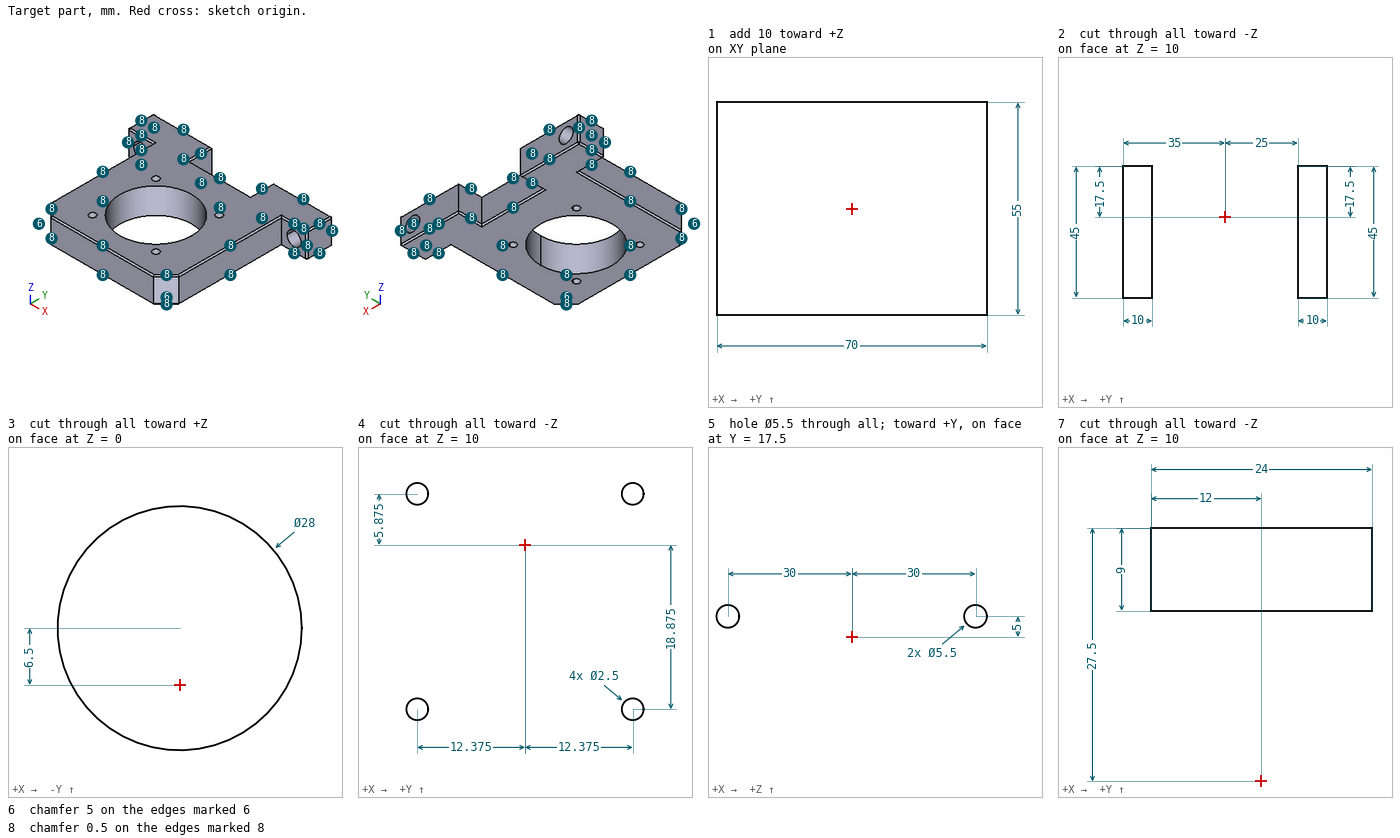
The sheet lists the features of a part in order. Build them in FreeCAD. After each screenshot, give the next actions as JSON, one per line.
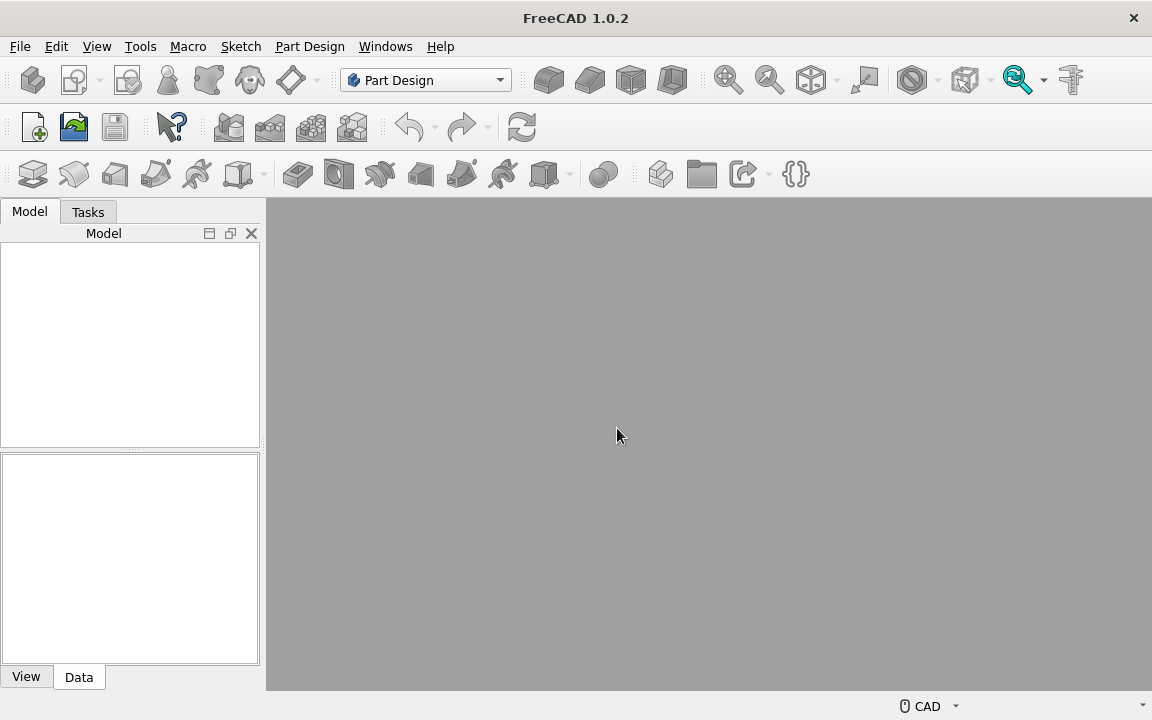
{"action": "left_click", "coordinate": [33, 128]}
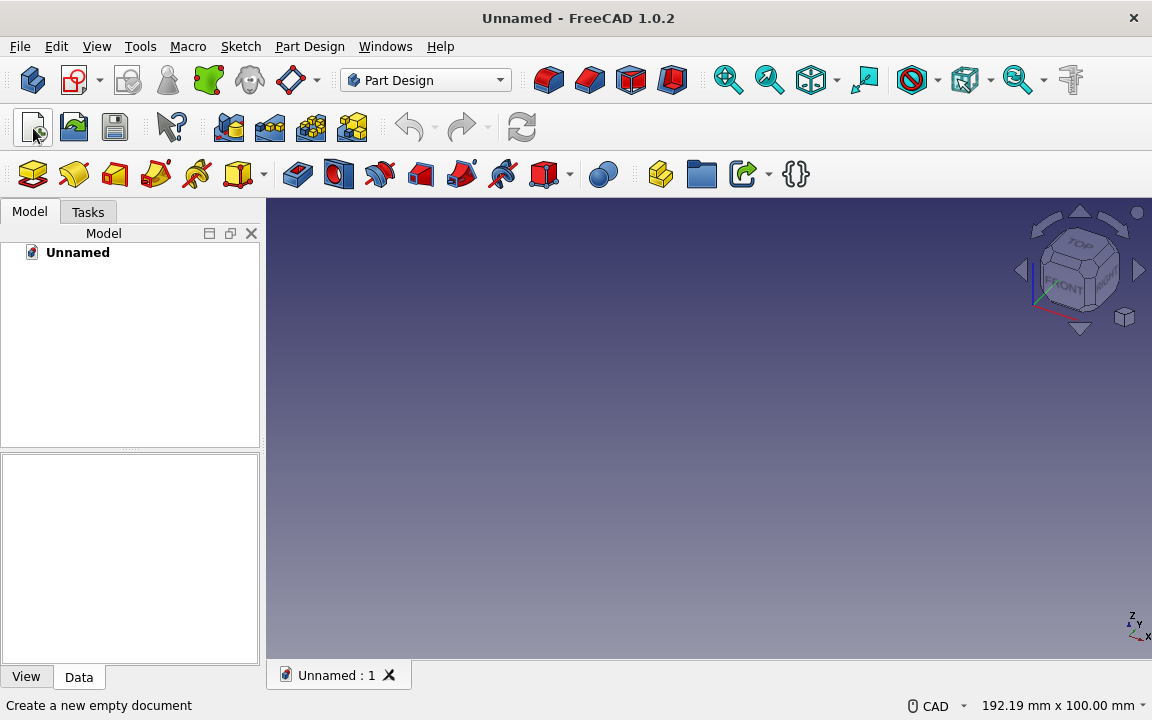
{"action": "left_click", "coordinate": [74, 80]}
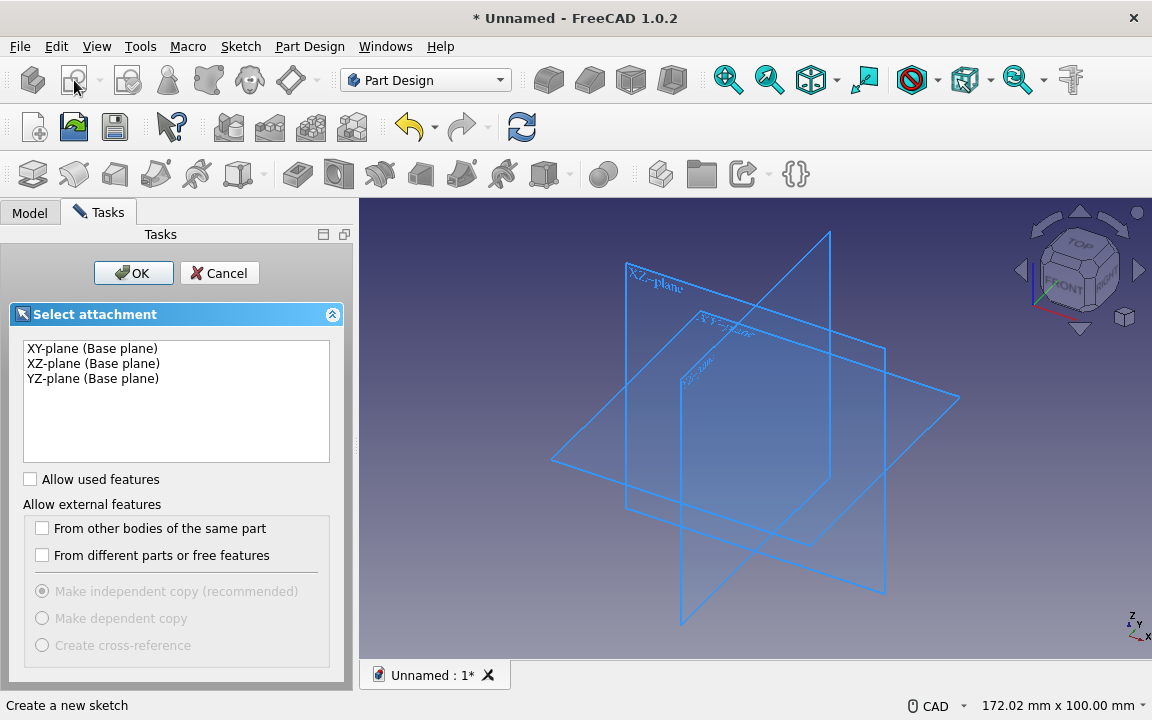
{"action": "left_click", "coordinate": [84, 348]}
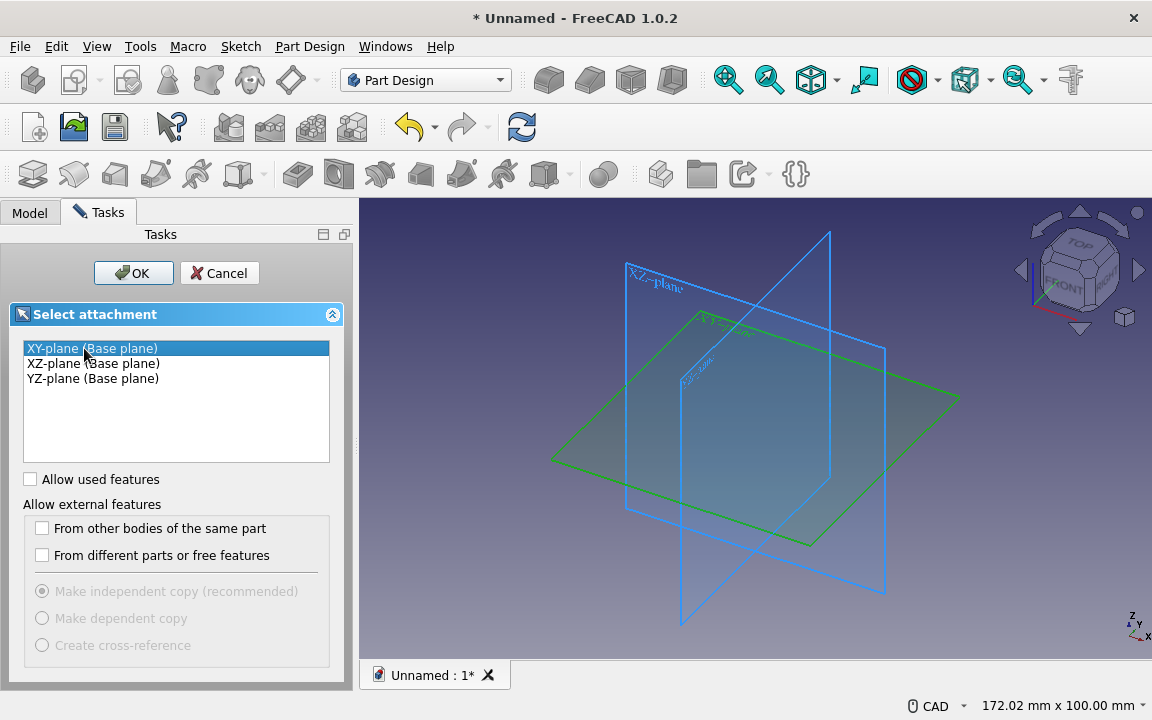
{"action": "left_click", "coordinate": [134, 273]}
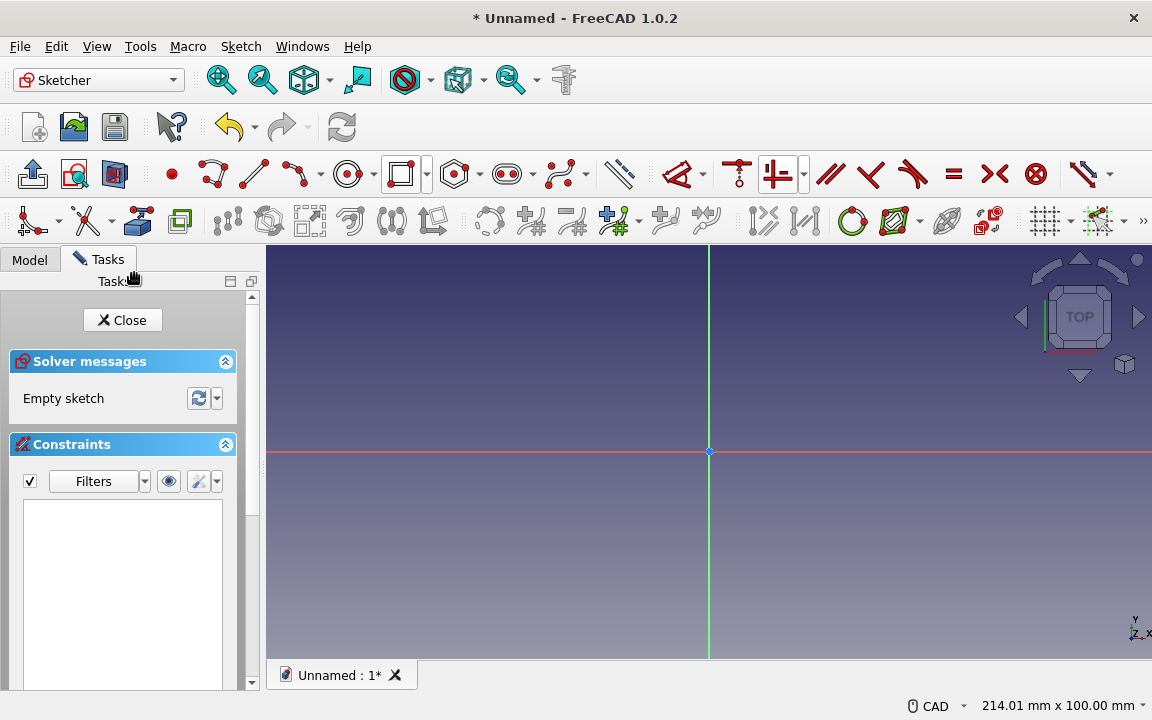
{"action": "left_click", "coordinate": [426, 174]}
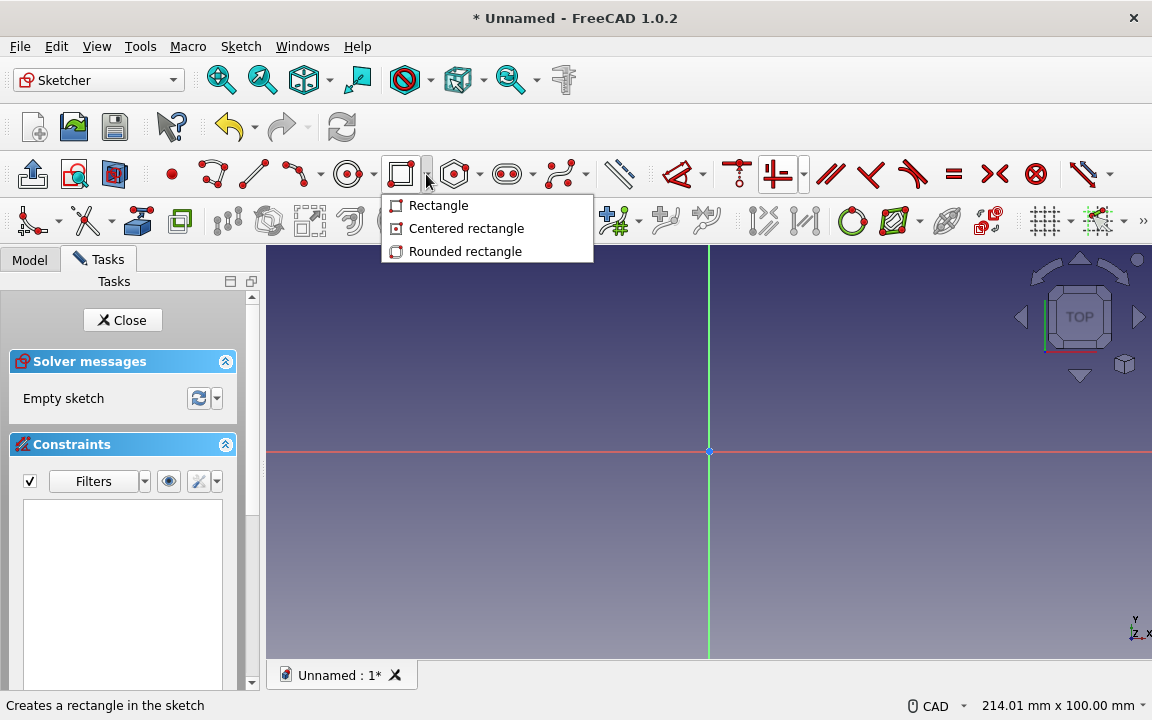
{"action": "left_click", "coordinate": [488, 228]}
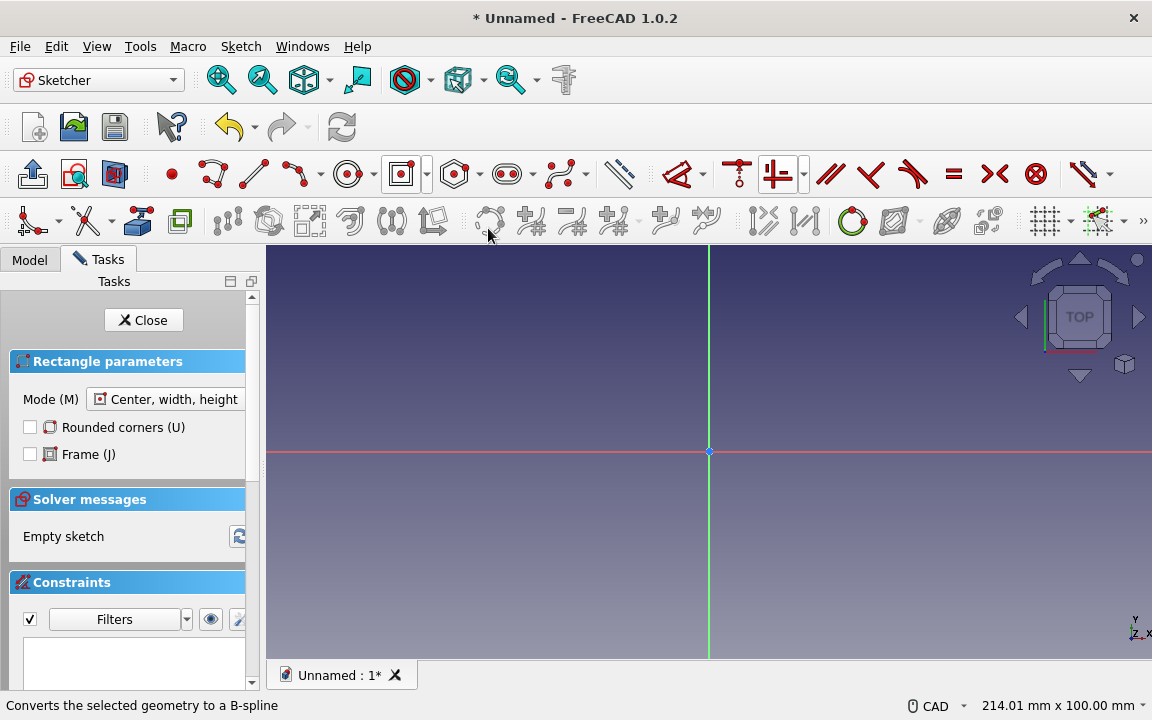
{"action": "left_click", "coordinate": [709, 452]}
{"action": "left_click", "coordinate": [854, 338]}
{"action": "key", "text": "Escape"}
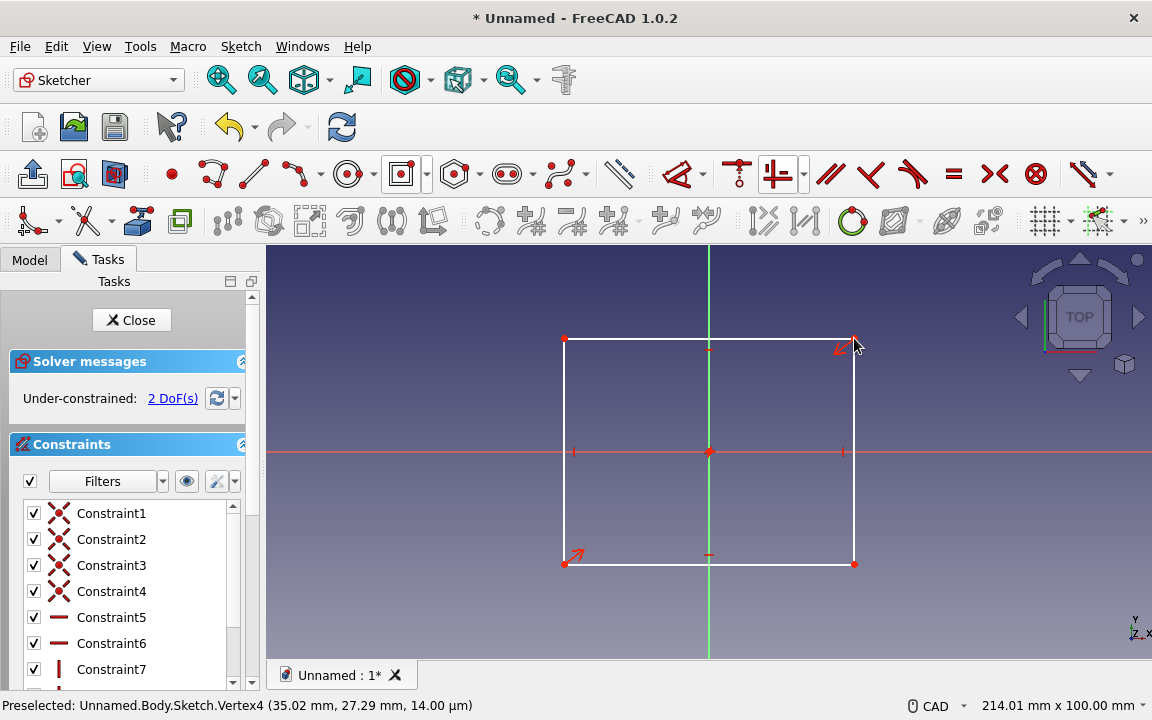
{"action": "left_click", "coordinate": [651, 565]}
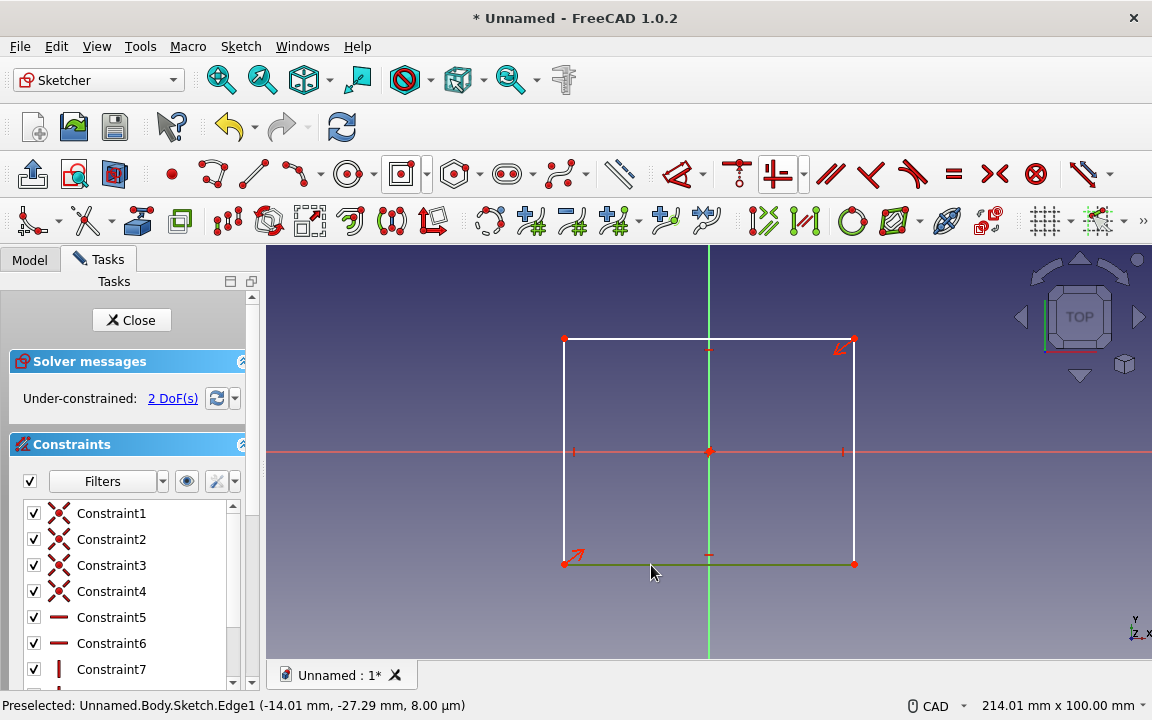
{"action": "key", "text": "l"}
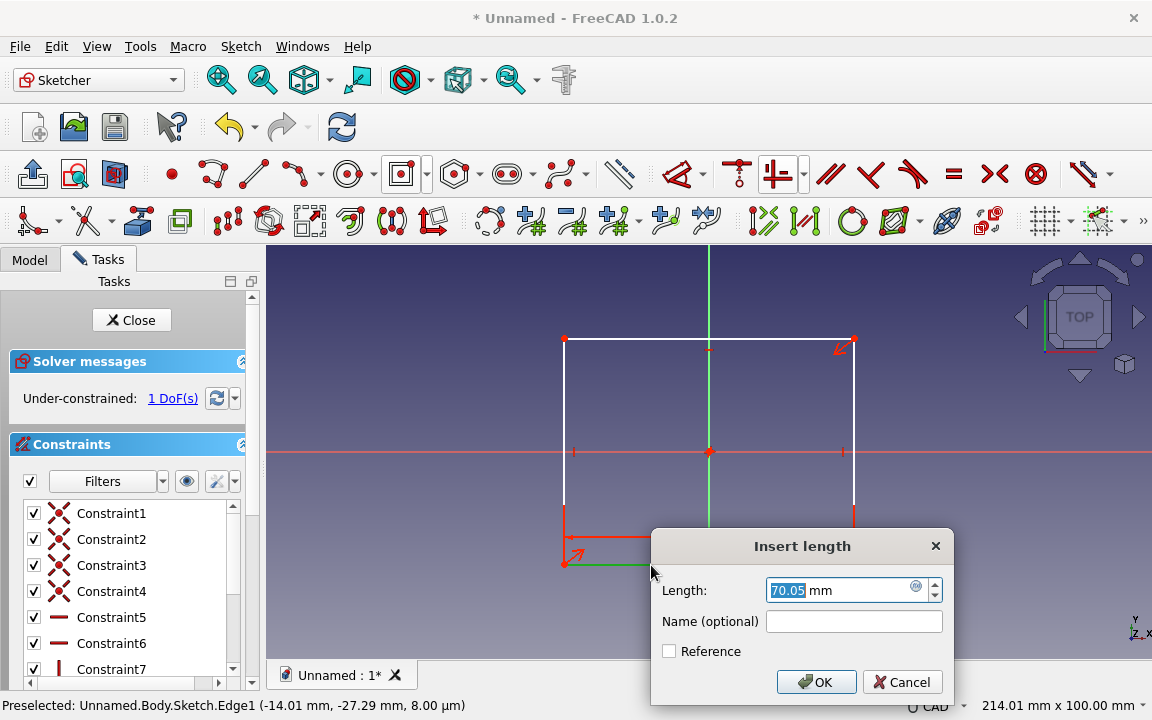
{"action": "type", "text": "70"}
{"action": "key", "text": "Return"}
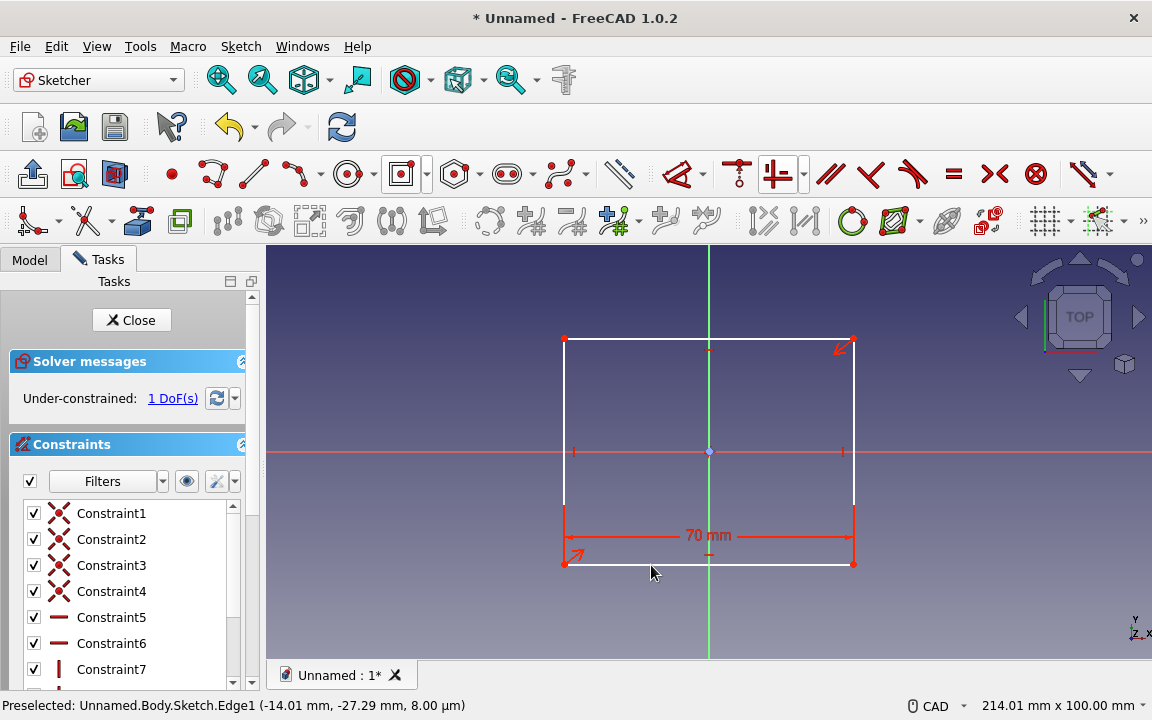
{"action": "left_click", "coordinate": [854, 497]}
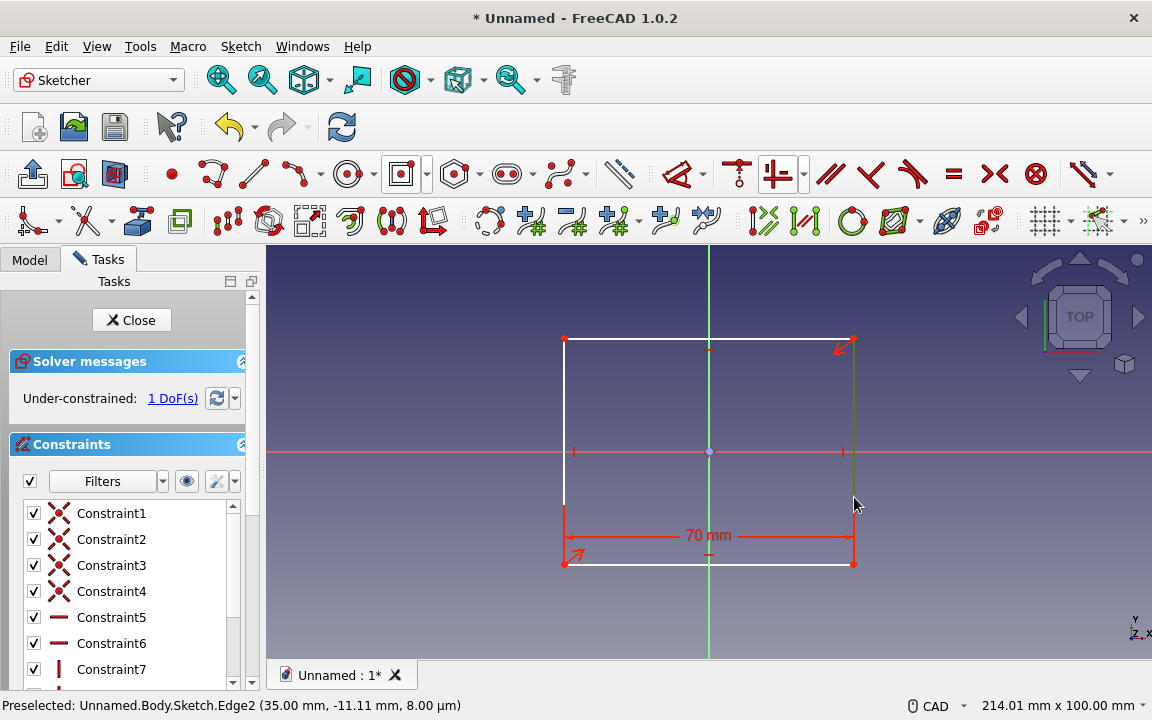
{"action": "key", "text": "i"}